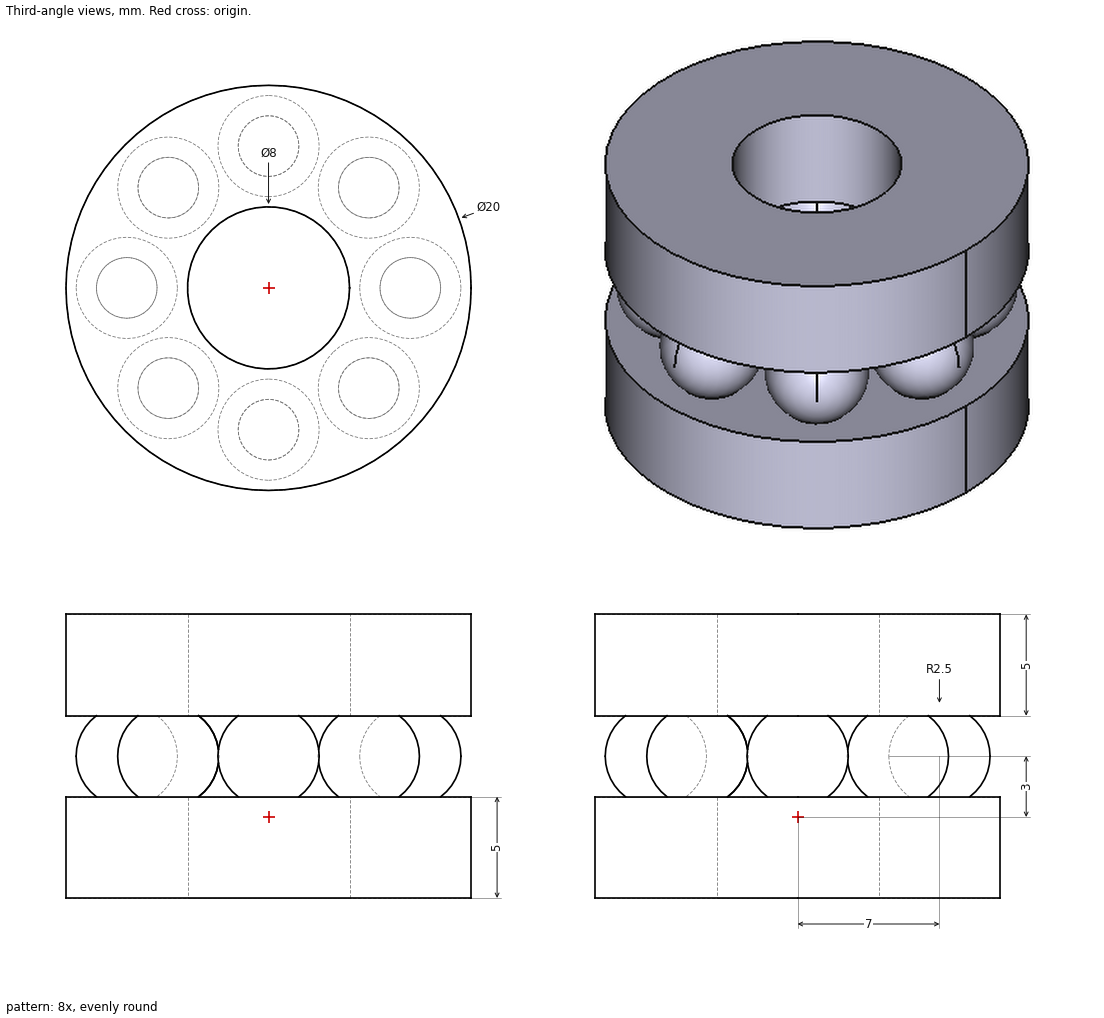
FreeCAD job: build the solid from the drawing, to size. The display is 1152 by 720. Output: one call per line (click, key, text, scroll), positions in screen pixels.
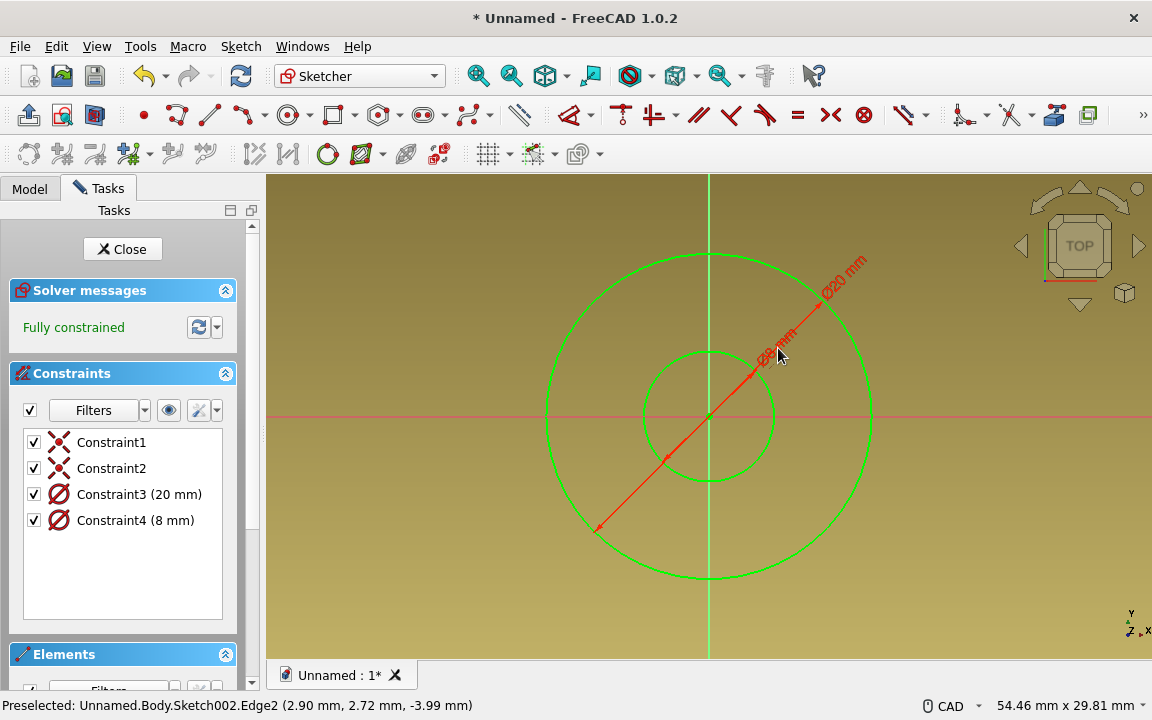
click(123, 249)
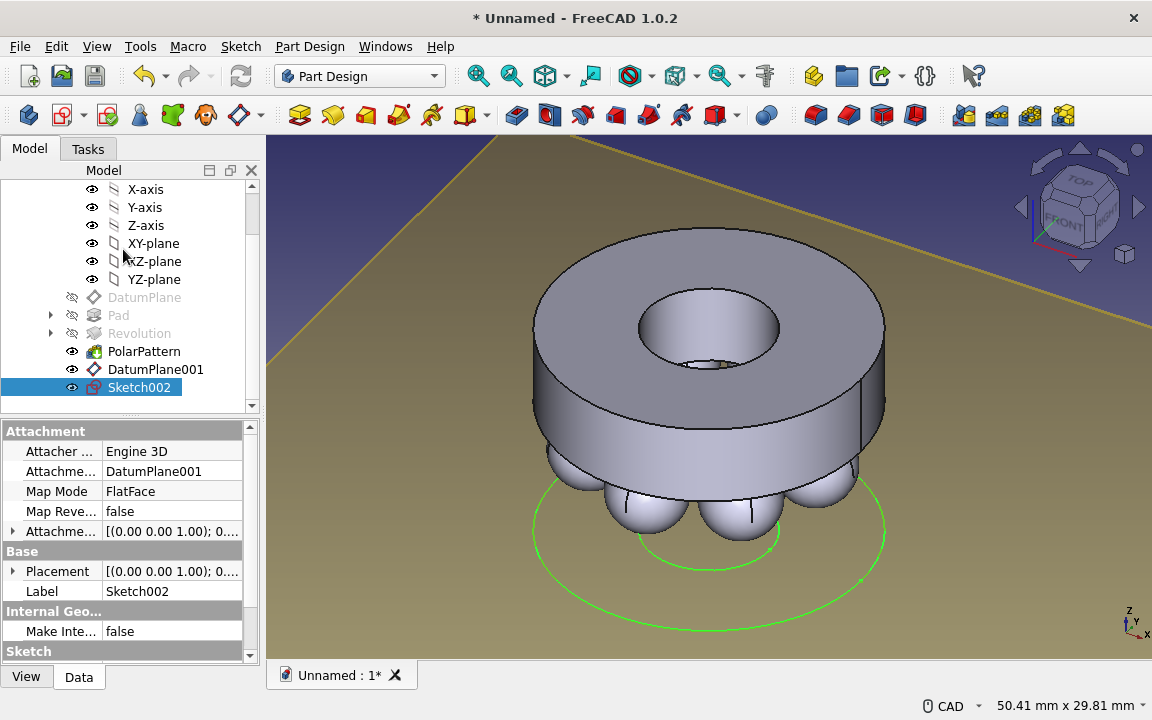
click(300, 116)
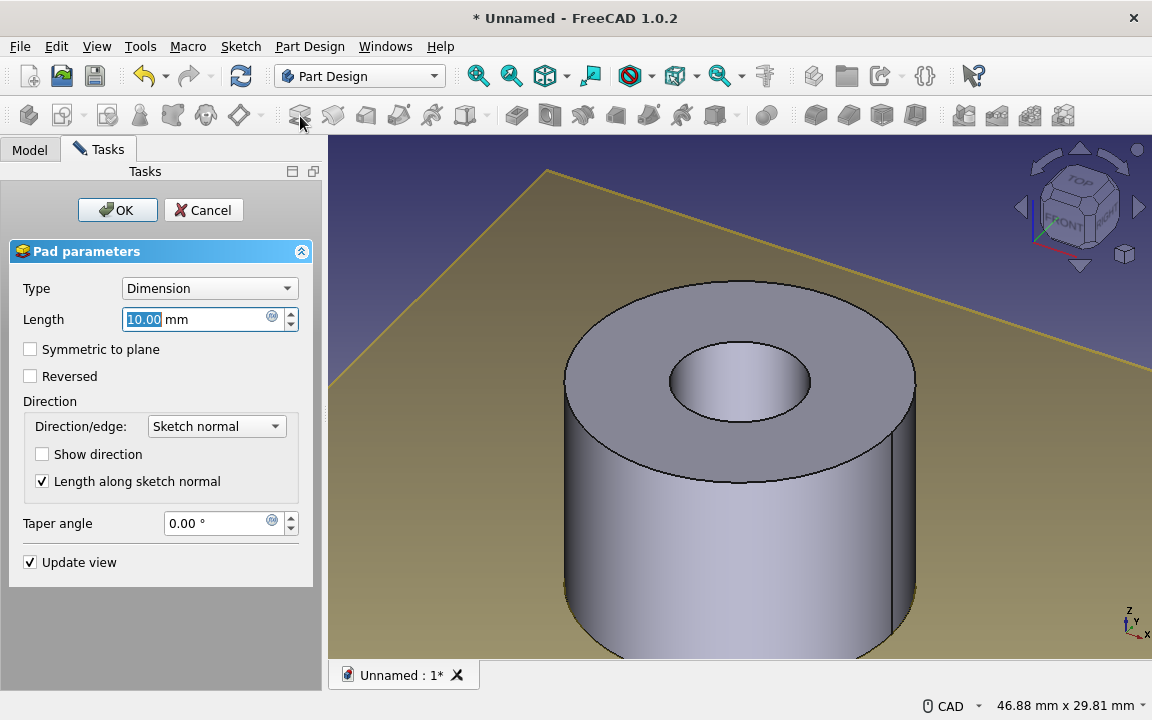
text(5)
key(Tab)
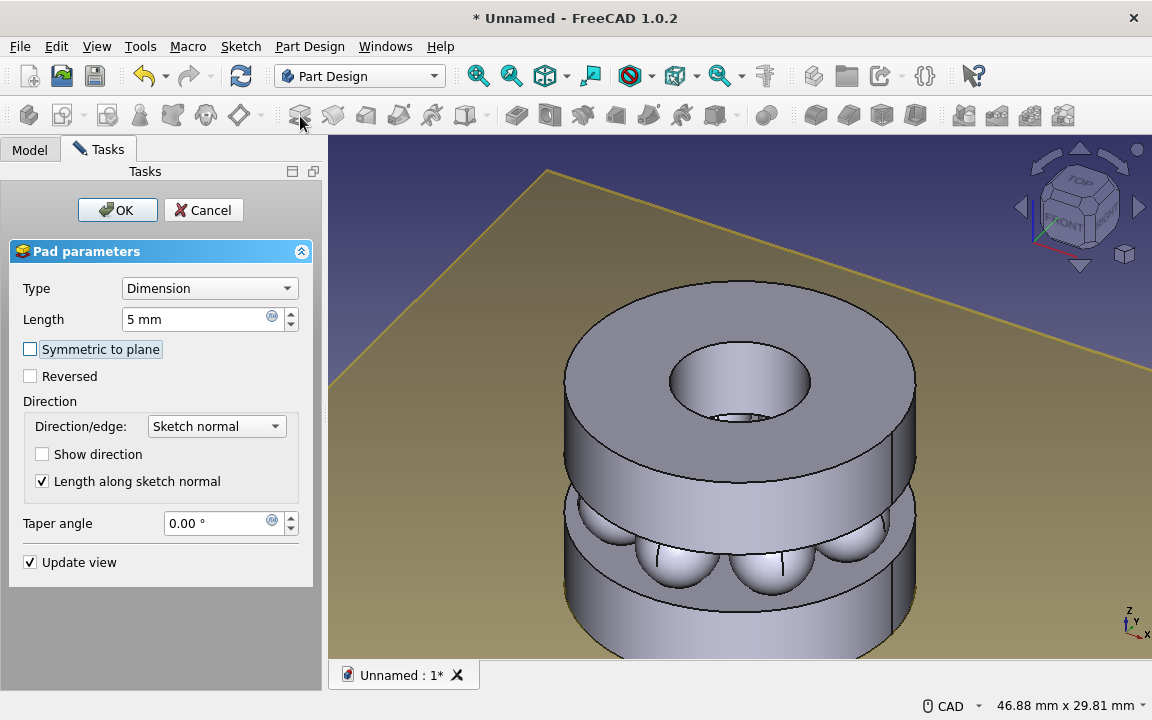
click(118, 210)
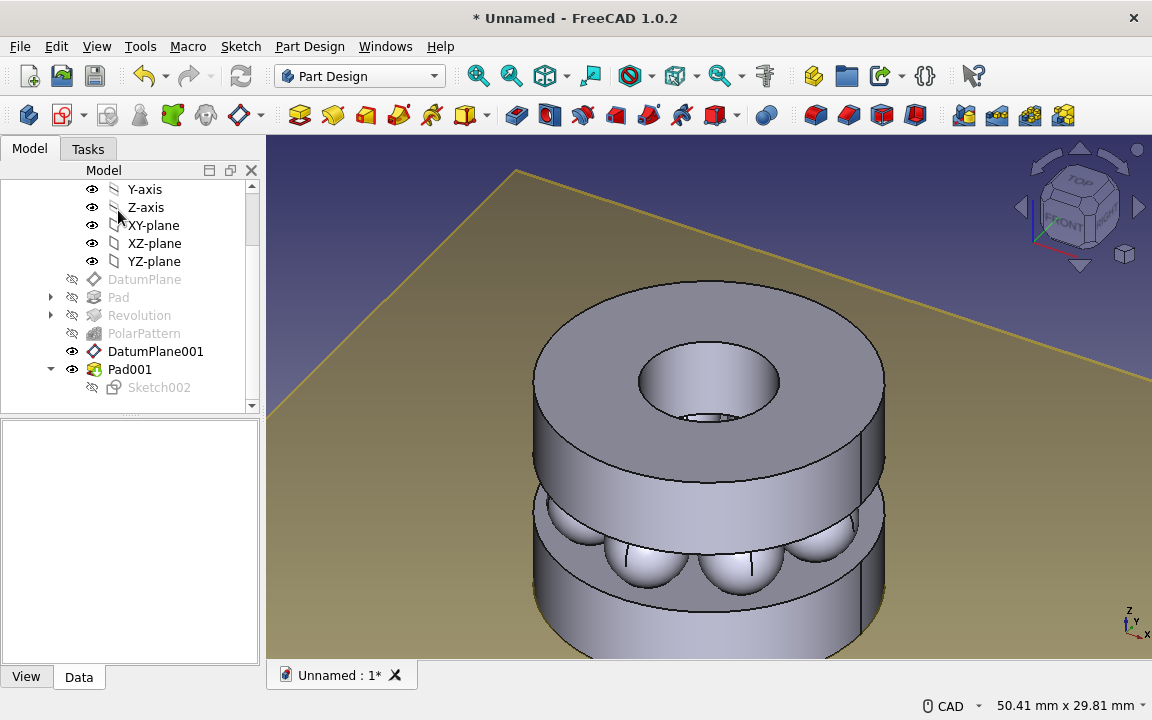
click(117, 351)
key(space)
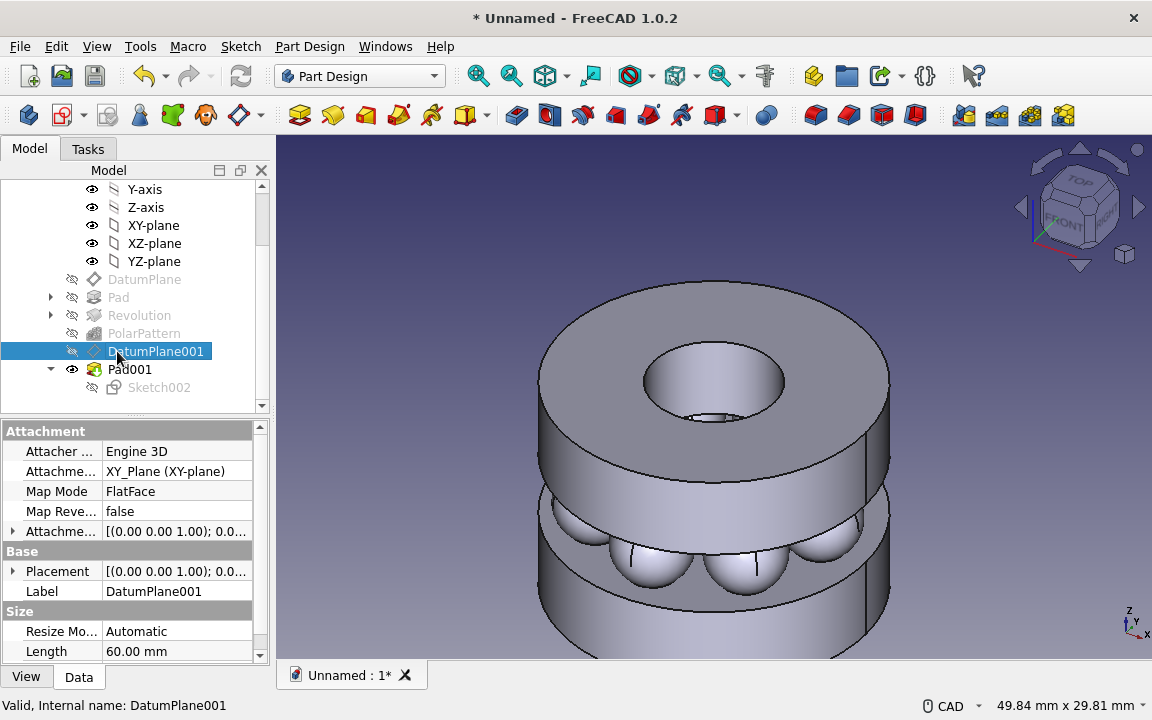
key(0)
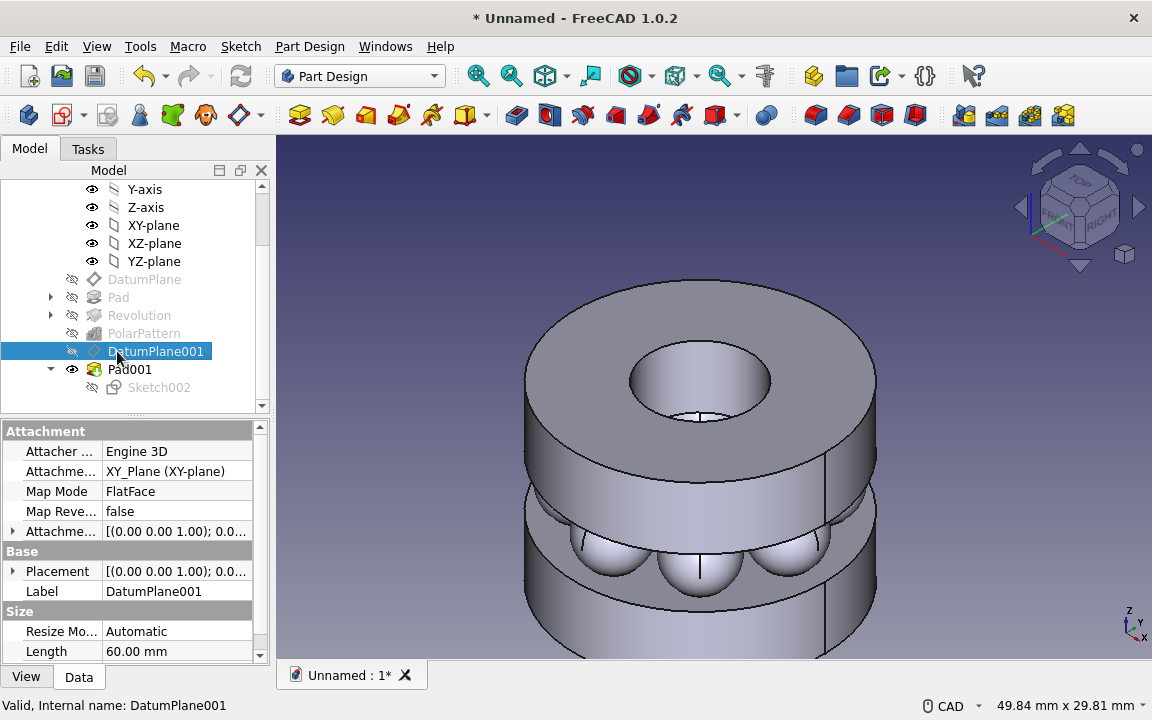
click(479, 76)